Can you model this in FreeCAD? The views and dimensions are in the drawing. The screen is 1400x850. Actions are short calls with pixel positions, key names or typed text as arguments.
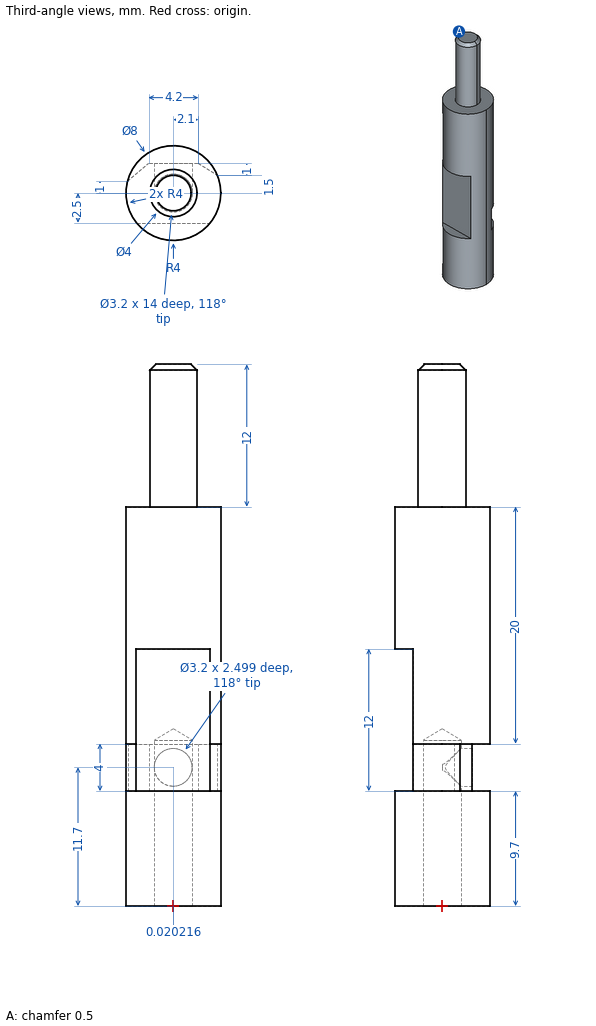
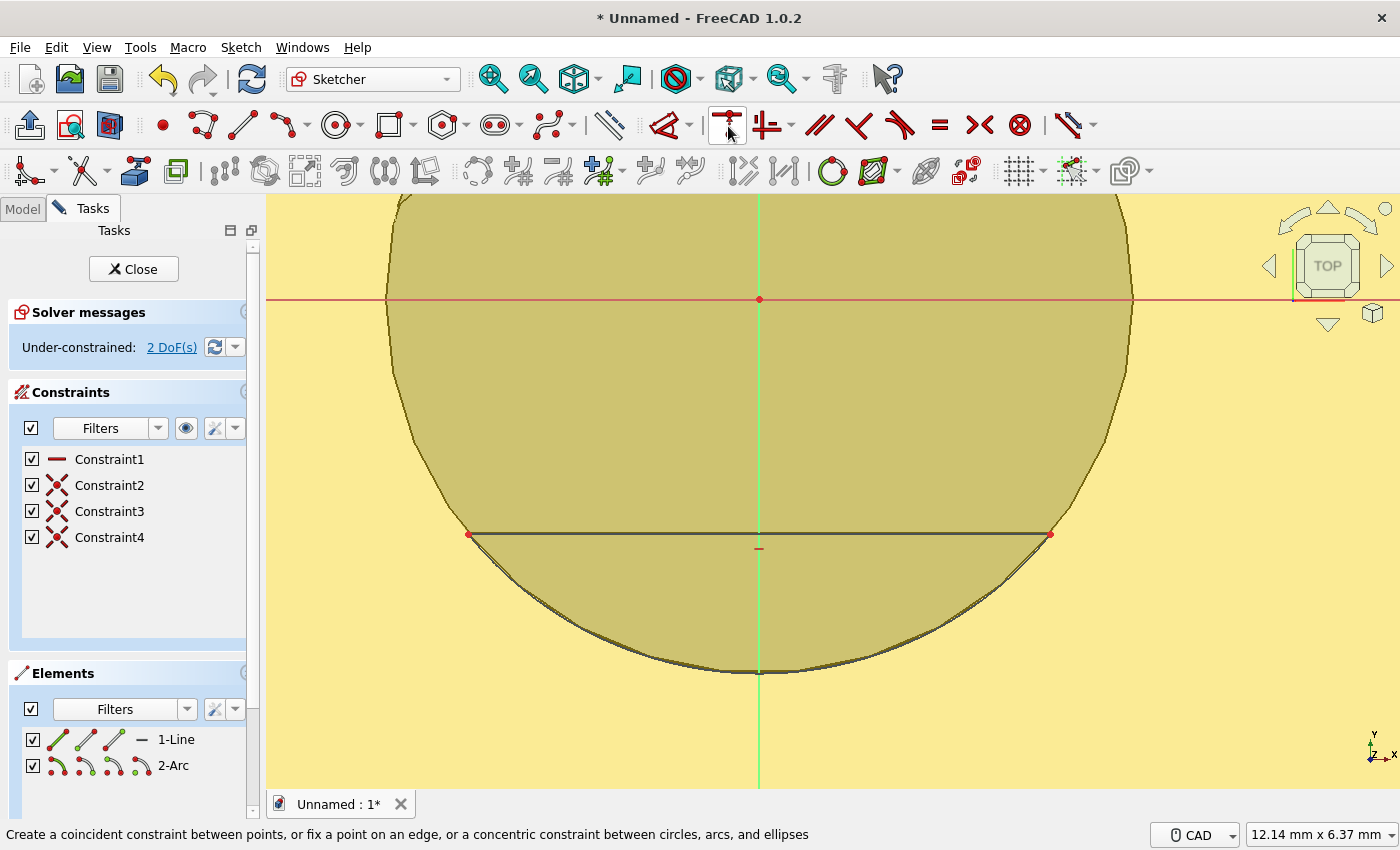
click(664, 126)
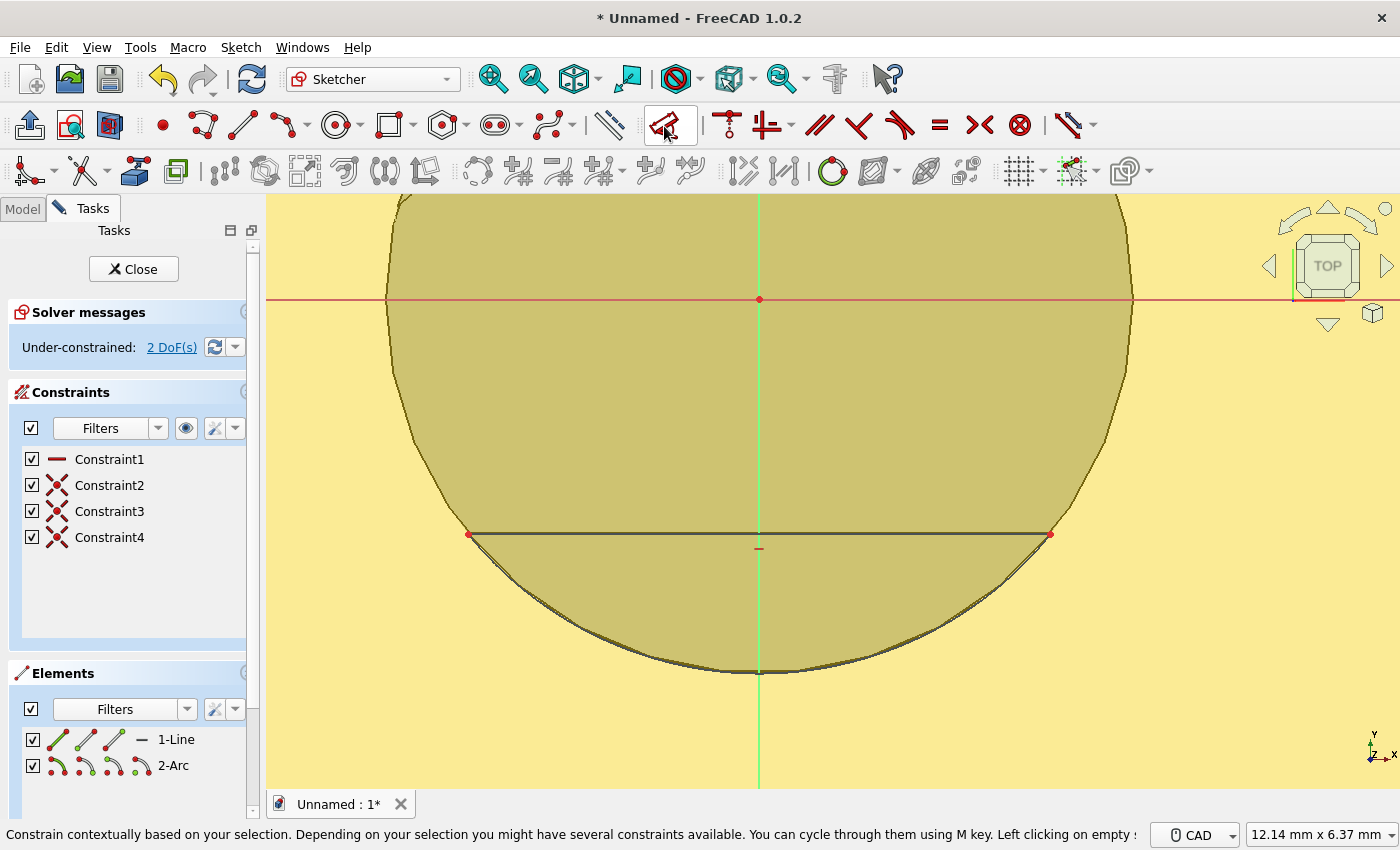
click(629, 650)
click(618, 680)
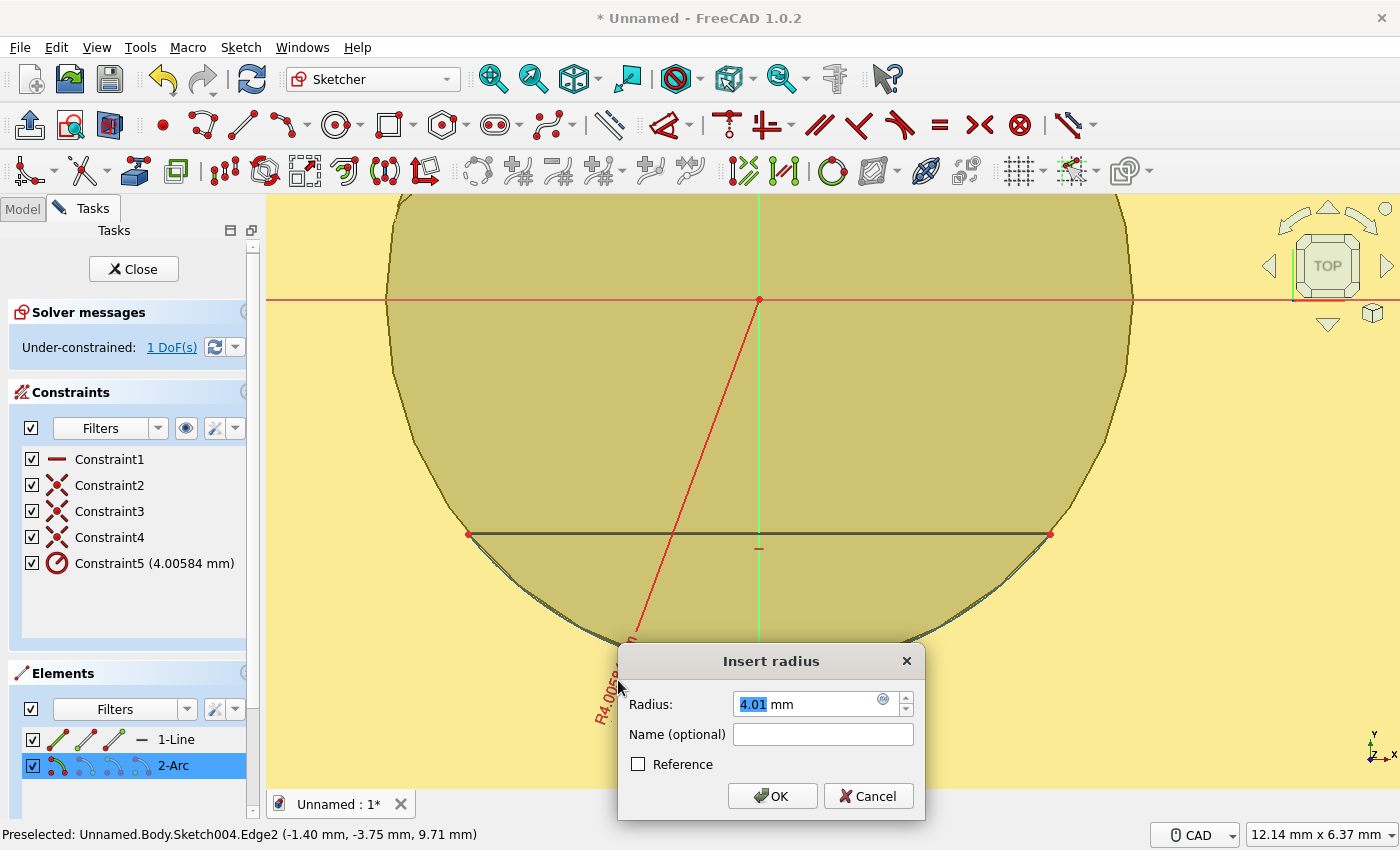
text(4)
key(Return)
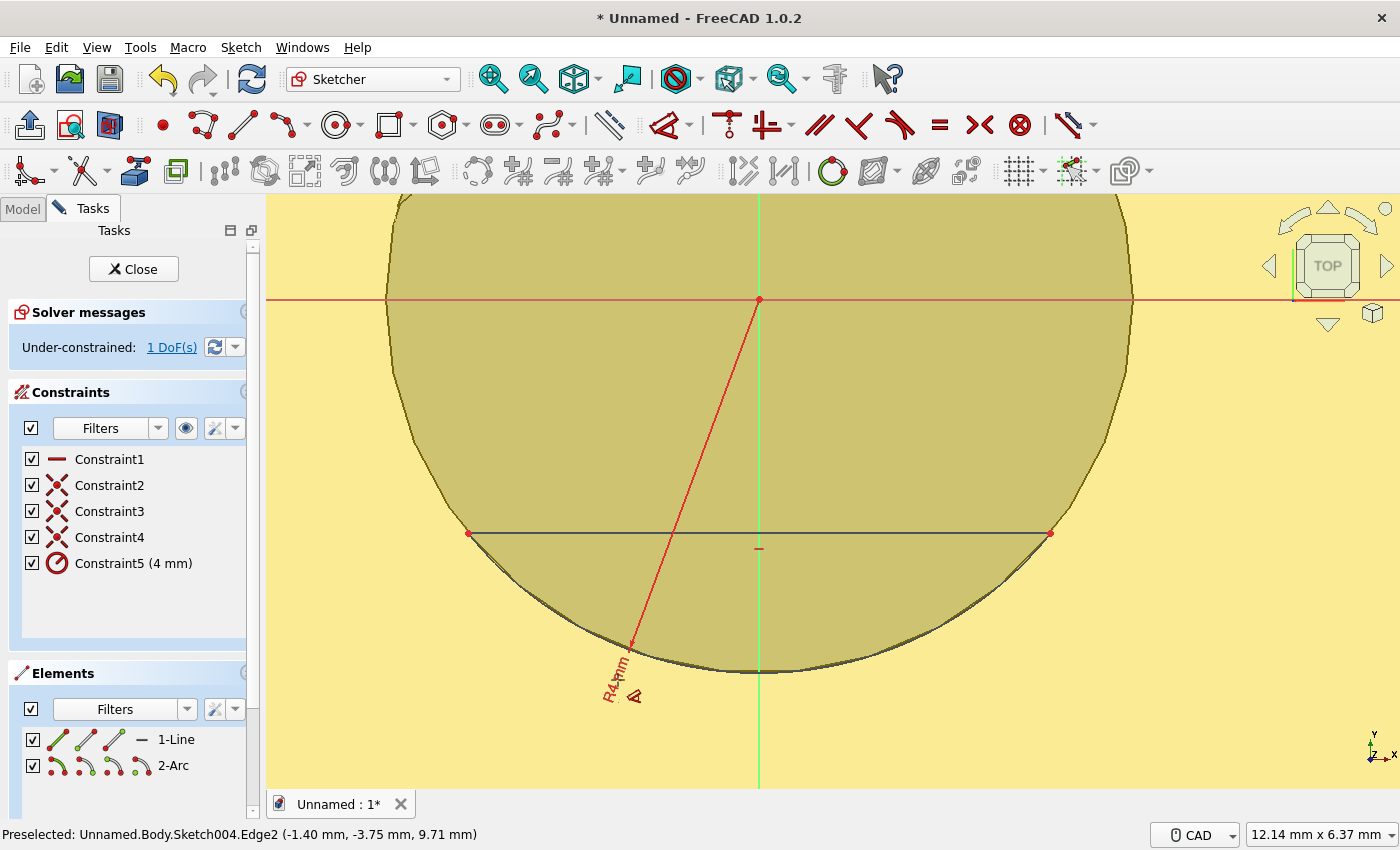
click(1051, 533)
click(1085, 416)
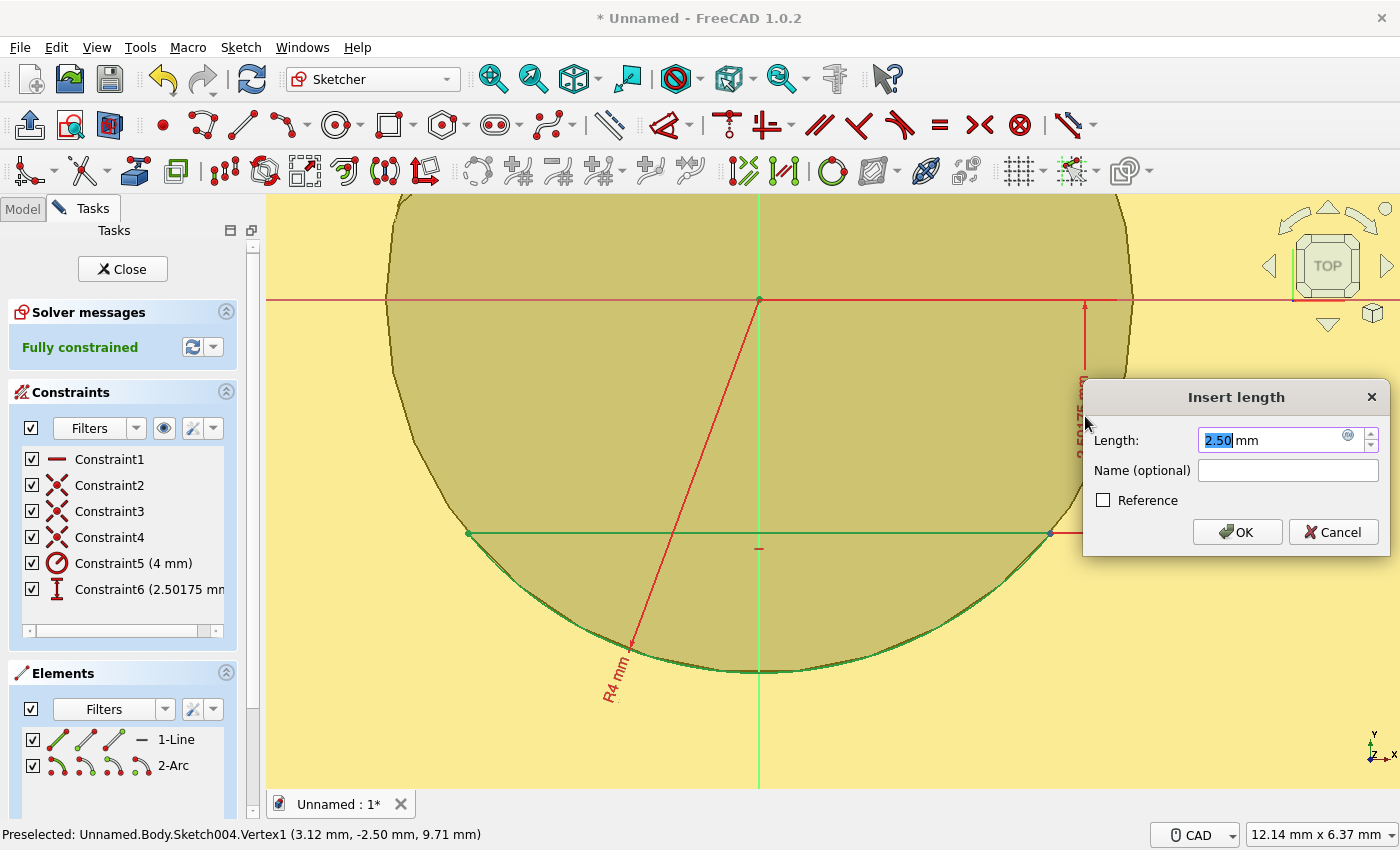
text(2.5)
key(Return)
key(Escape)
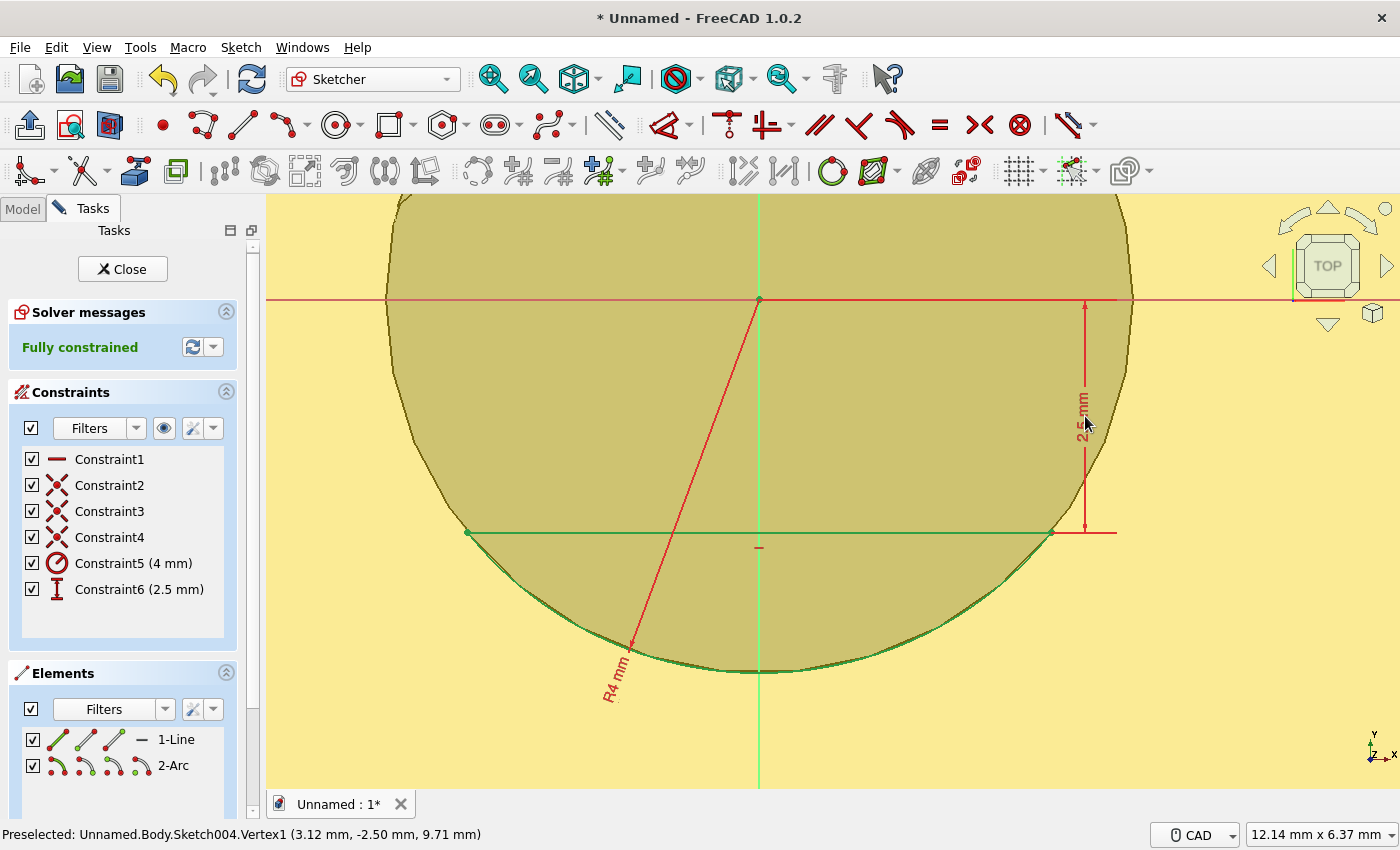
click(123, 269)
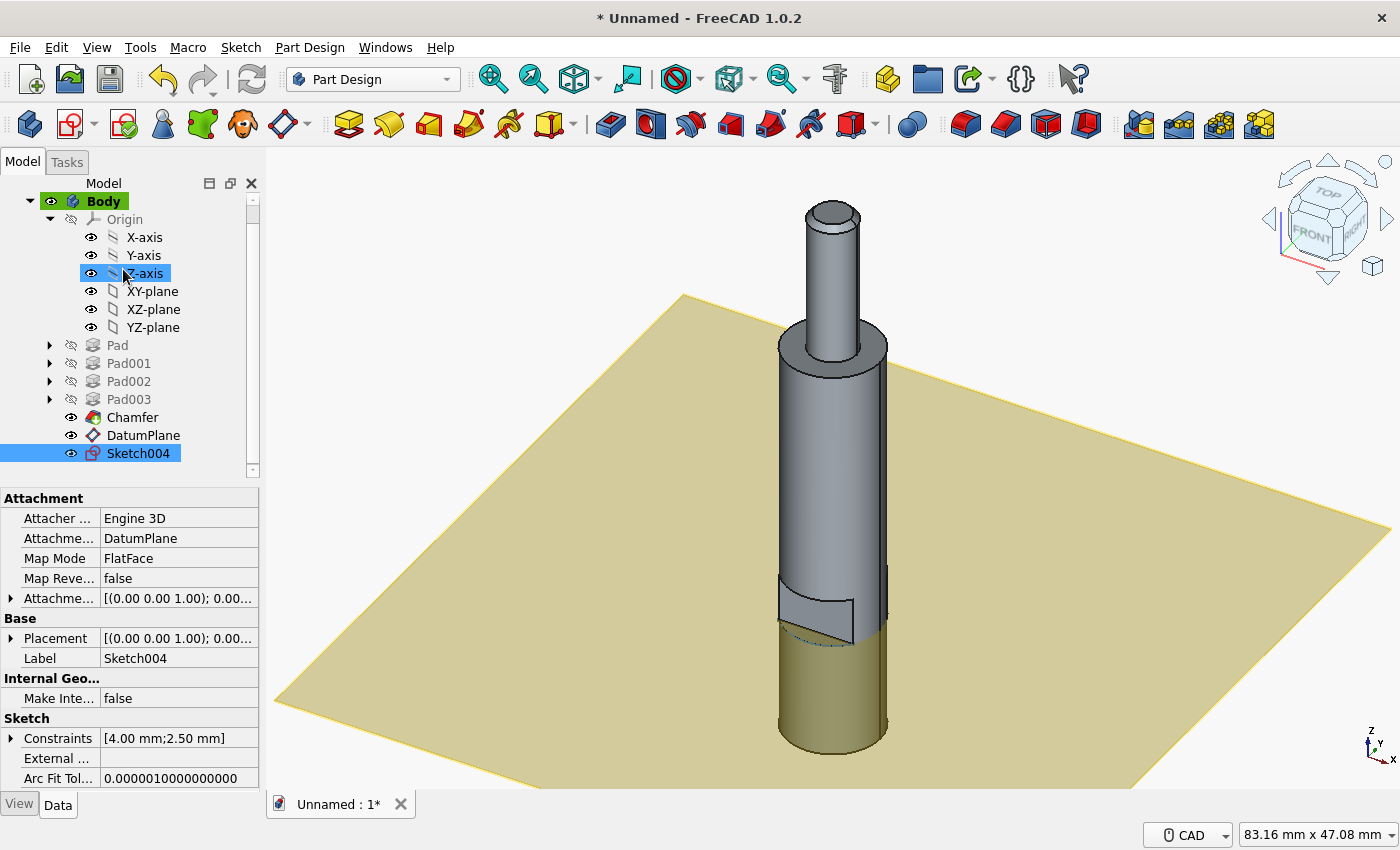
click(612, 124)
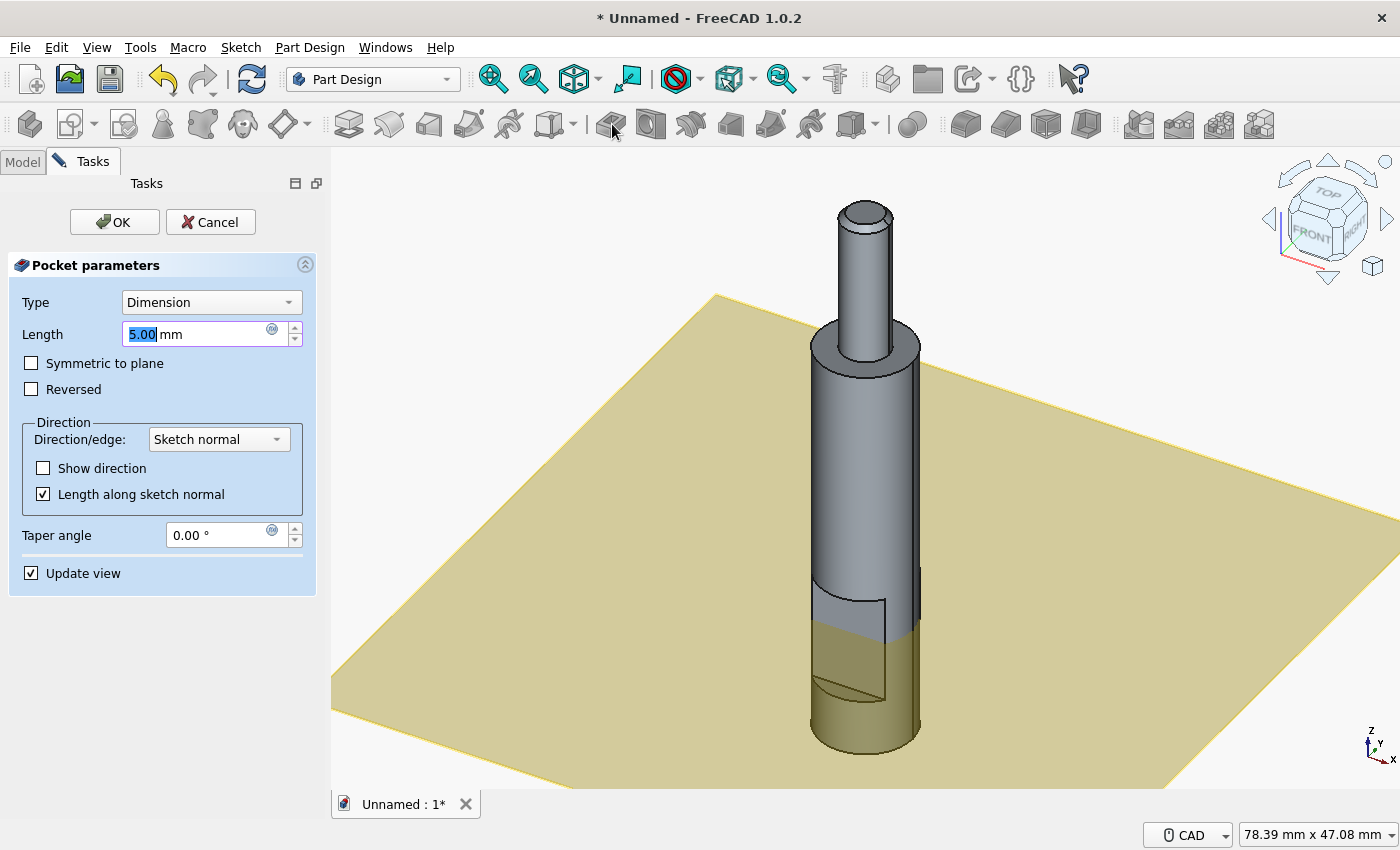
text(12)
key(Tab)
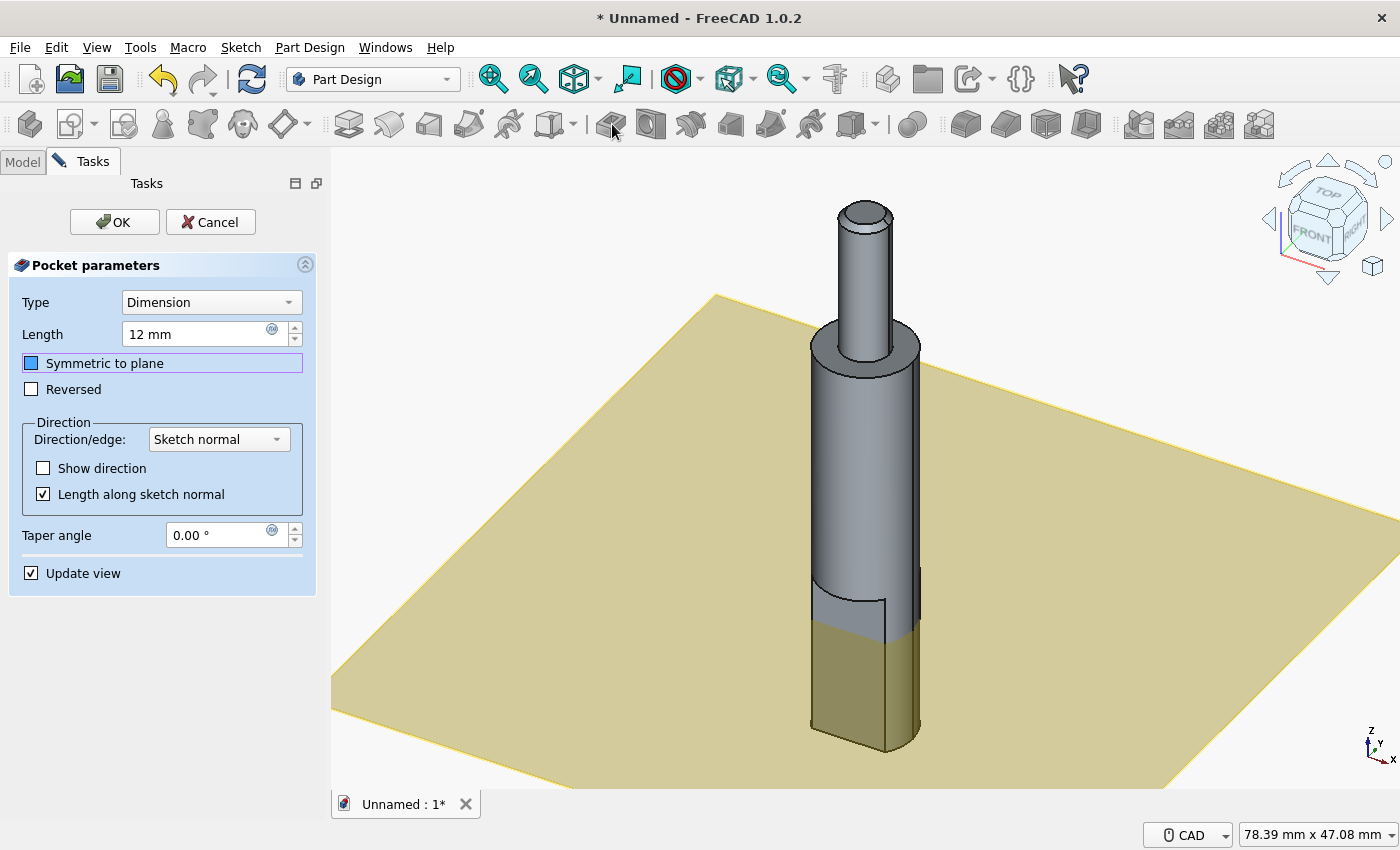
click(30, 389)